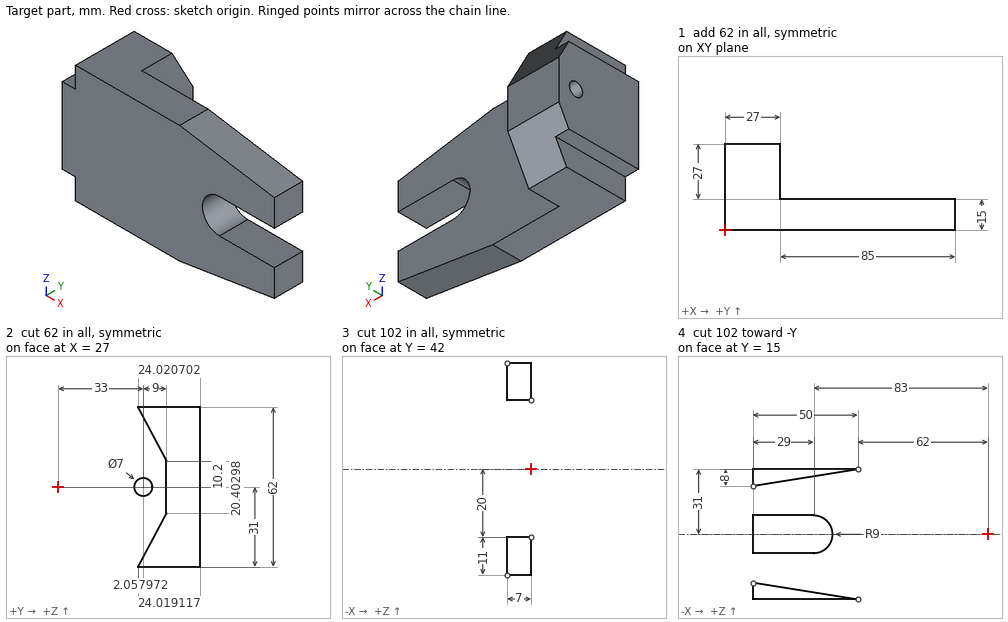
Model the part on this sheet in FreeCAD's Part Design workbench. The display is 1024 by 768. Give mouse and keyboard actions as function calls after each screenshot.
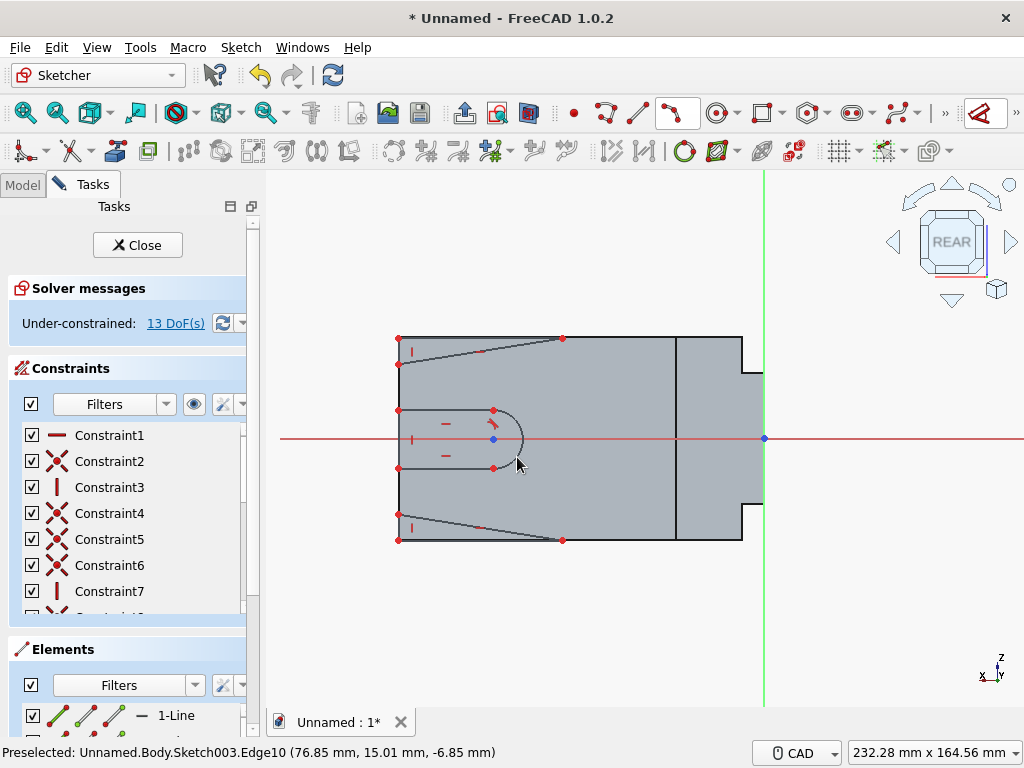
click(427, 469)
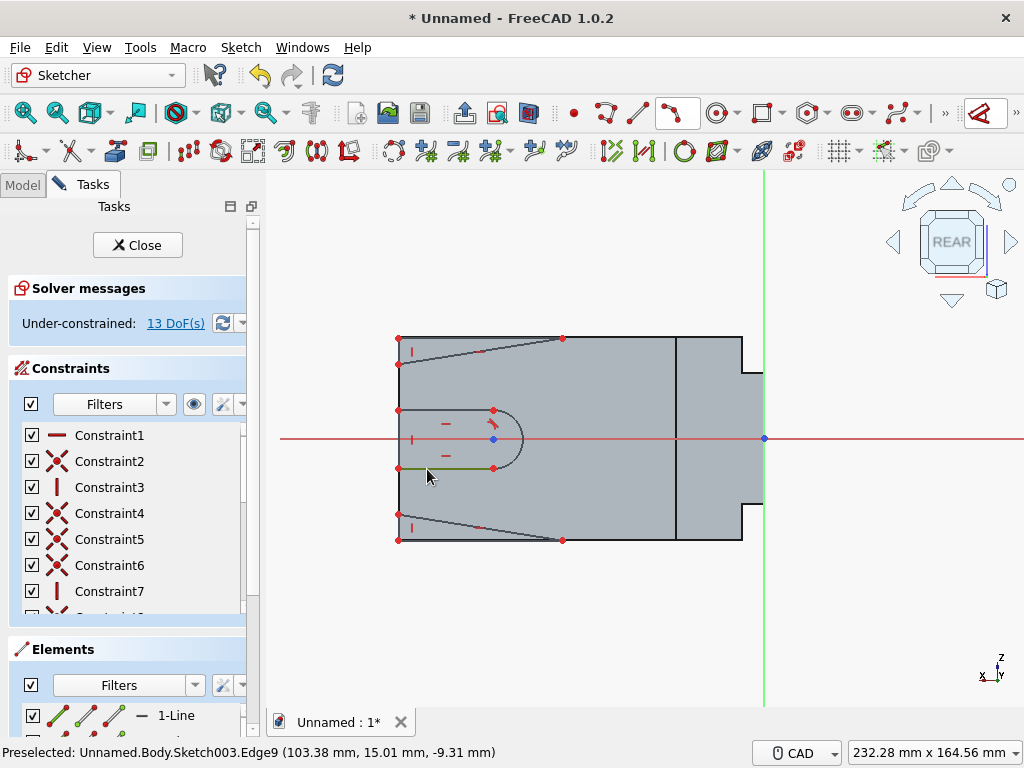
click(517, 457)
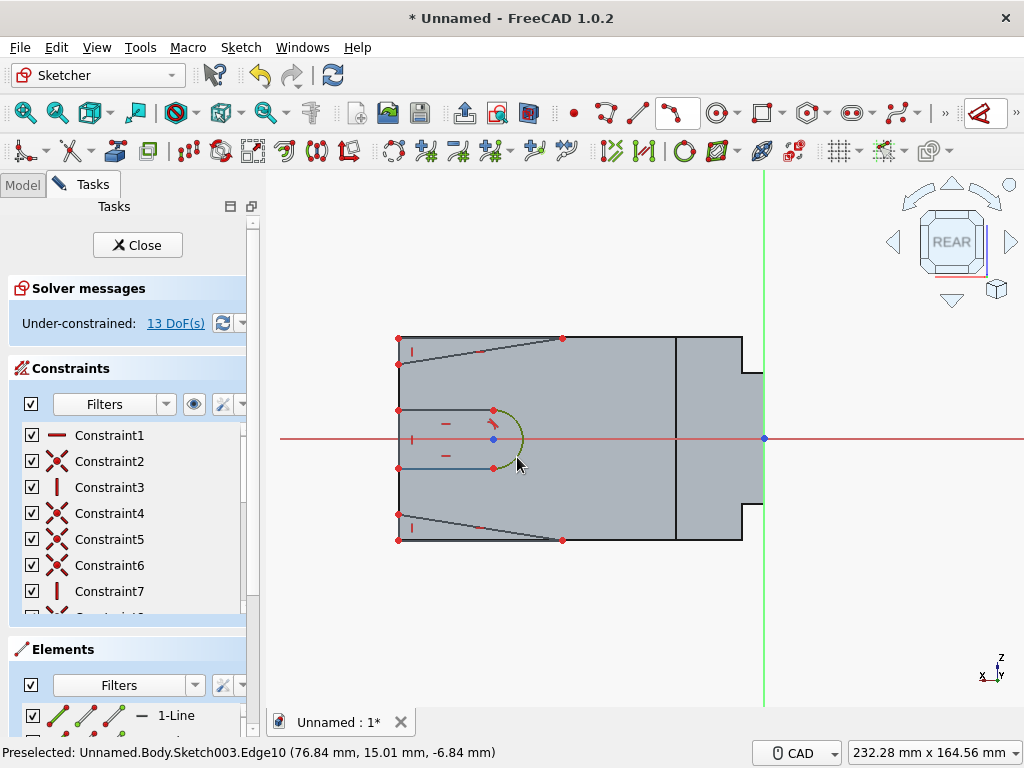
key(t)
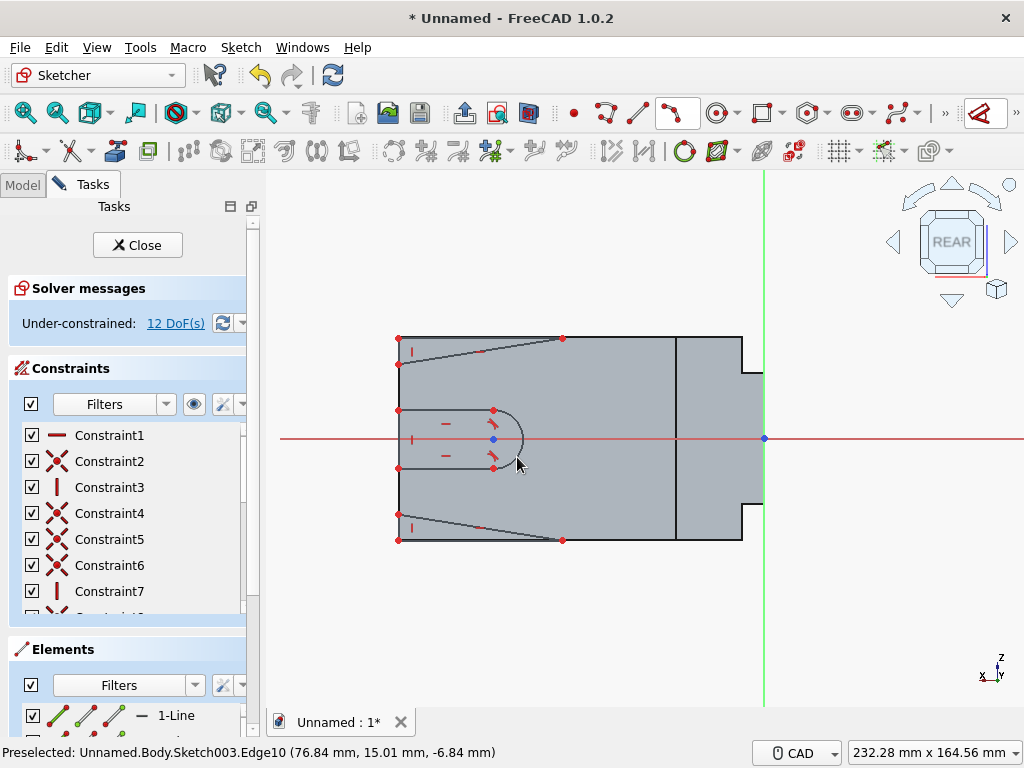
click(494, 439)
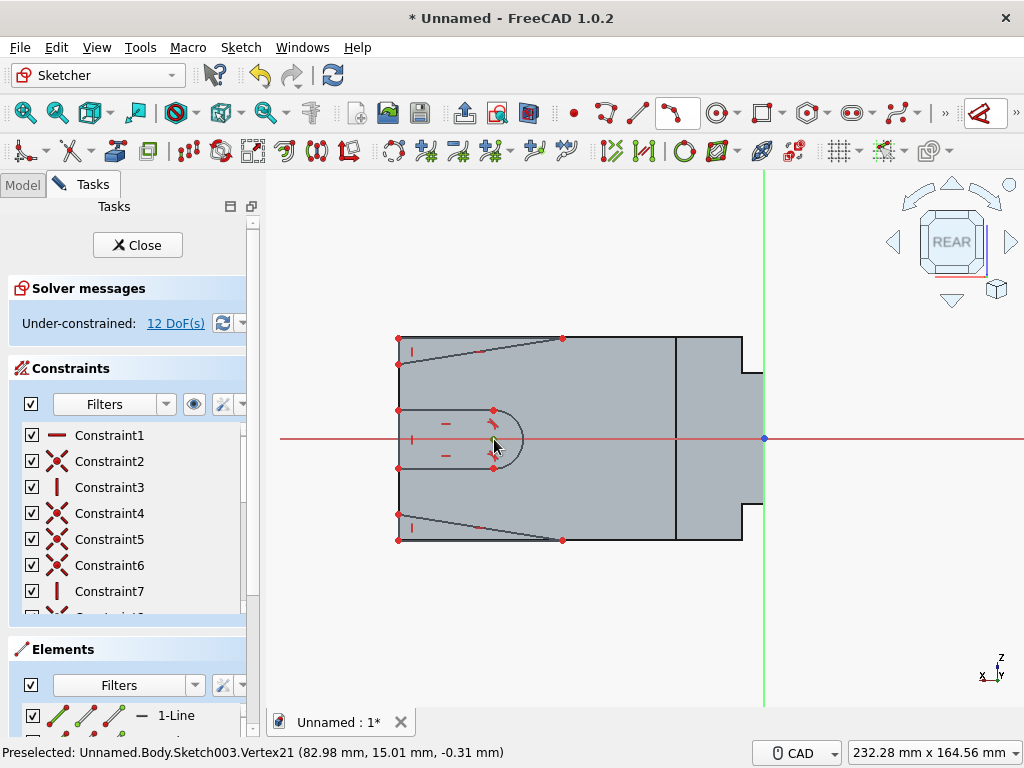
click(334, 439)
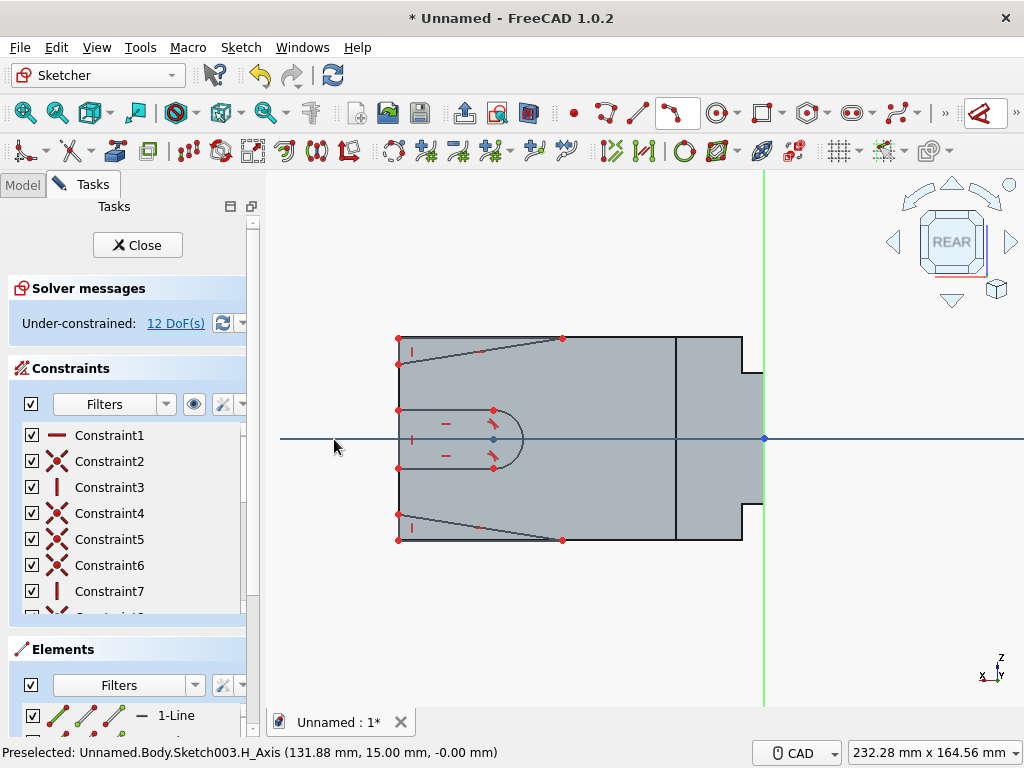
key(c)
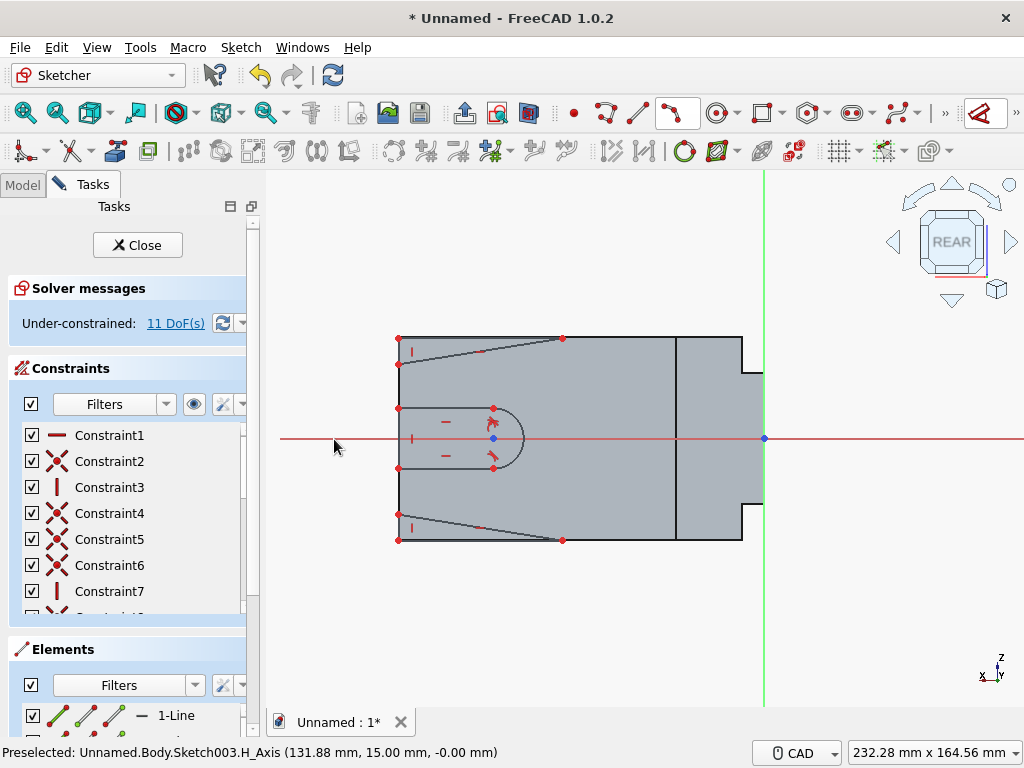
click(562, 338)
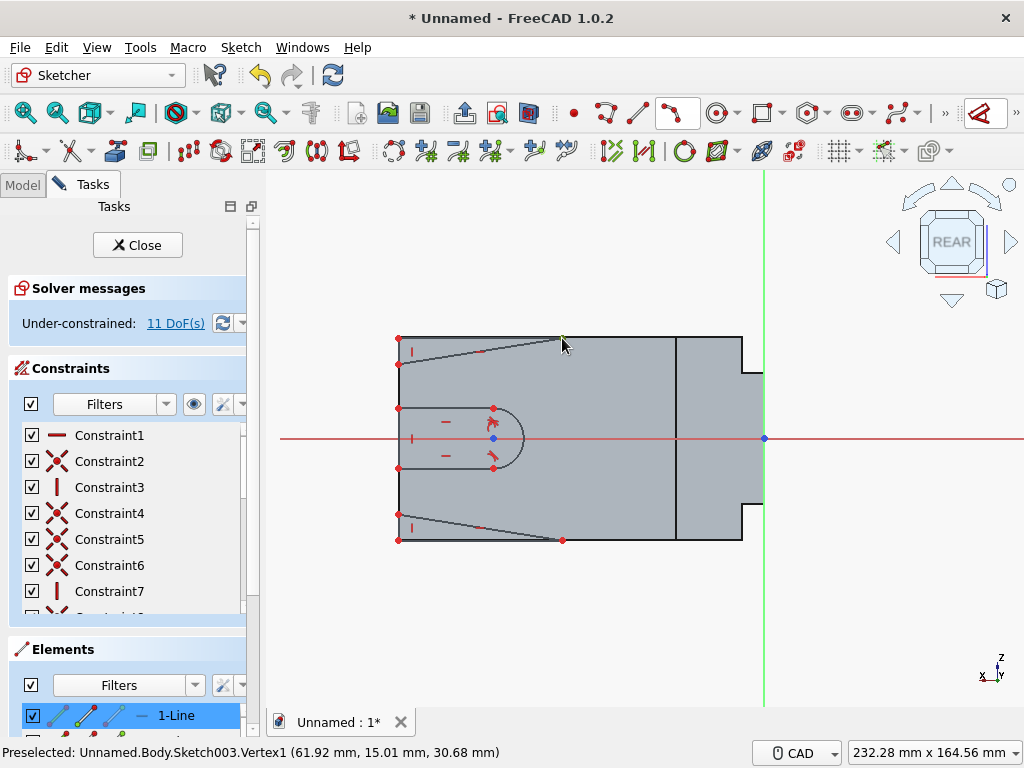
click(562, 541)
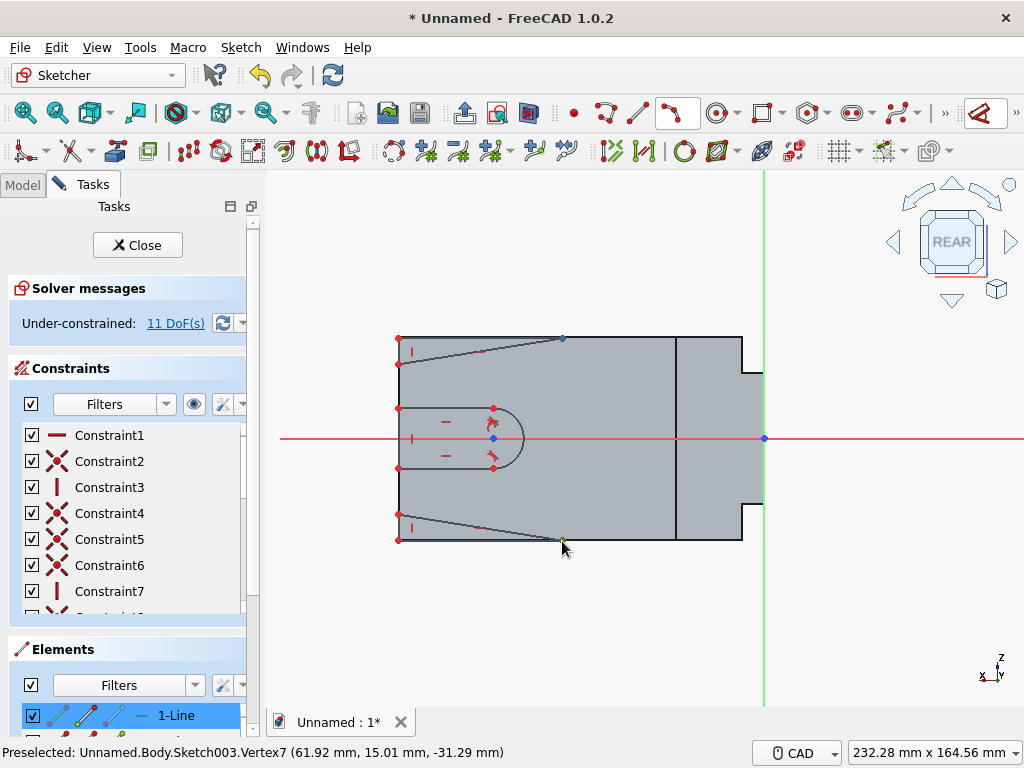
click(334, 439)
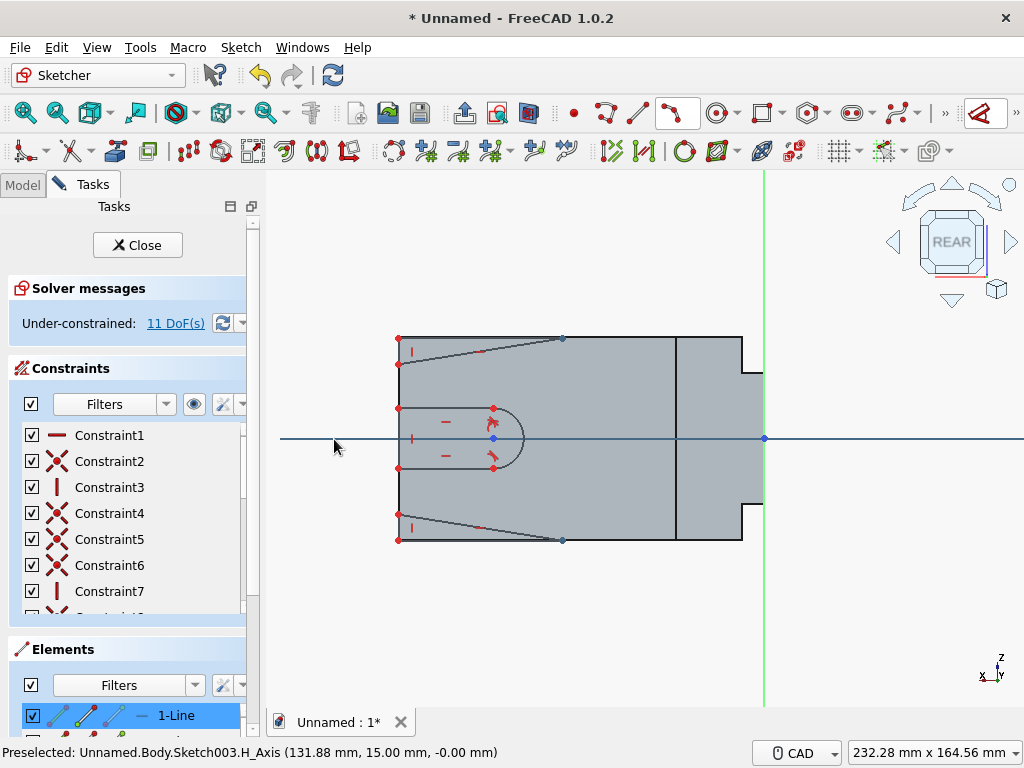
key(s)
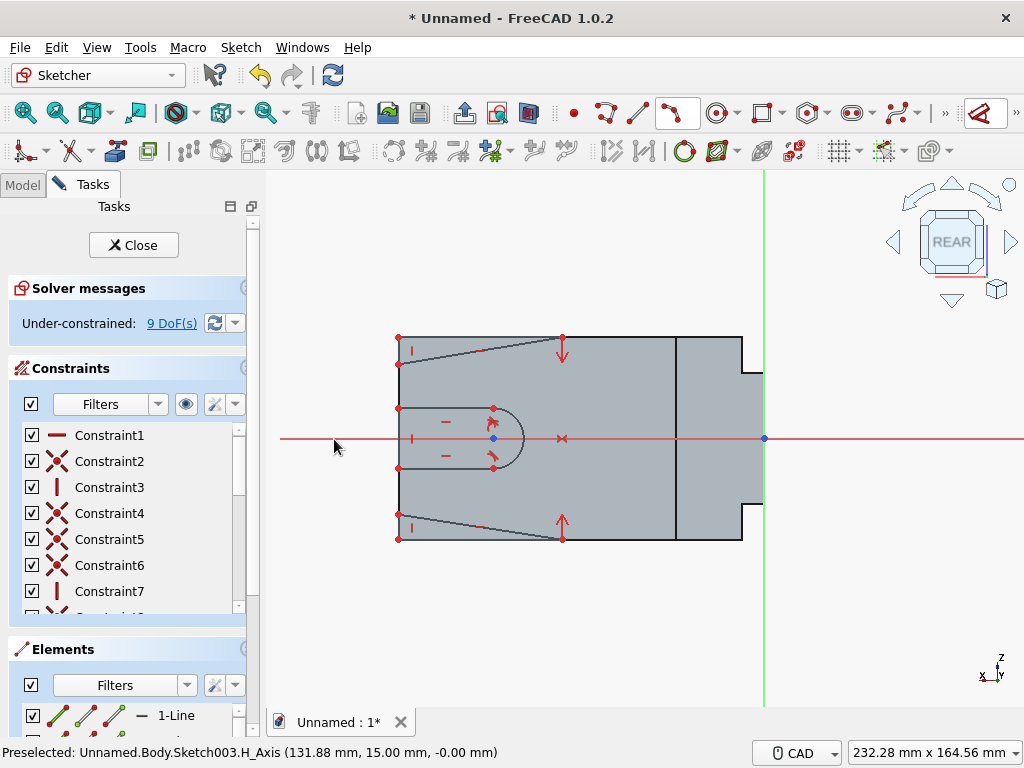
click(399, 364)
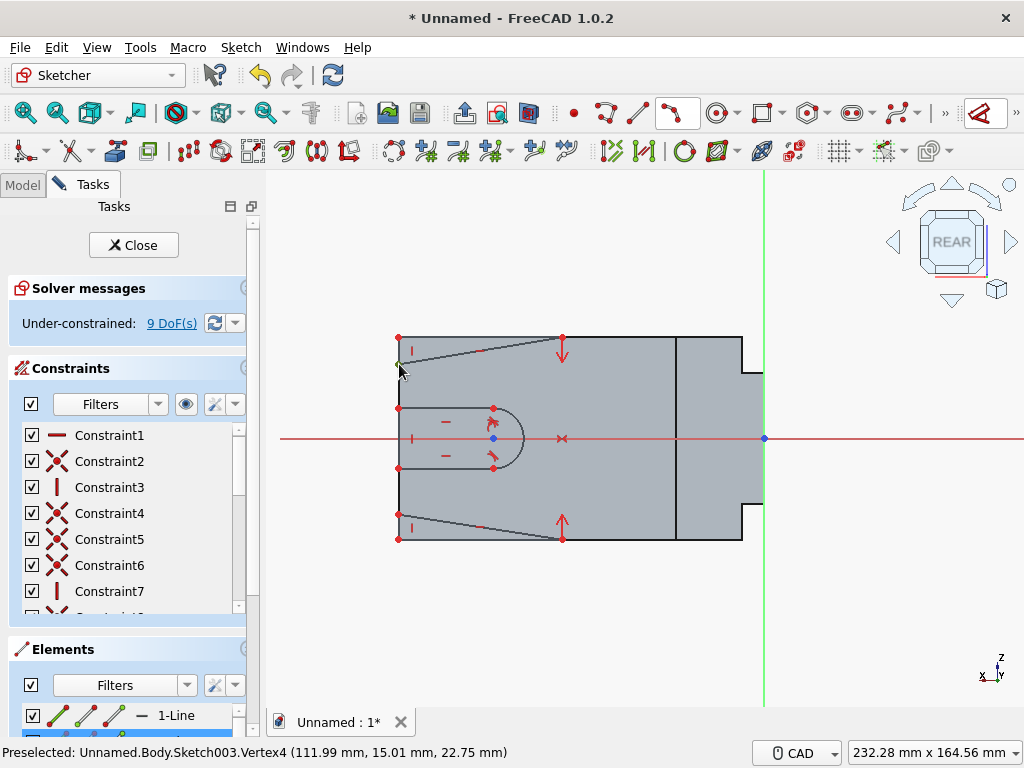
click(399, 515)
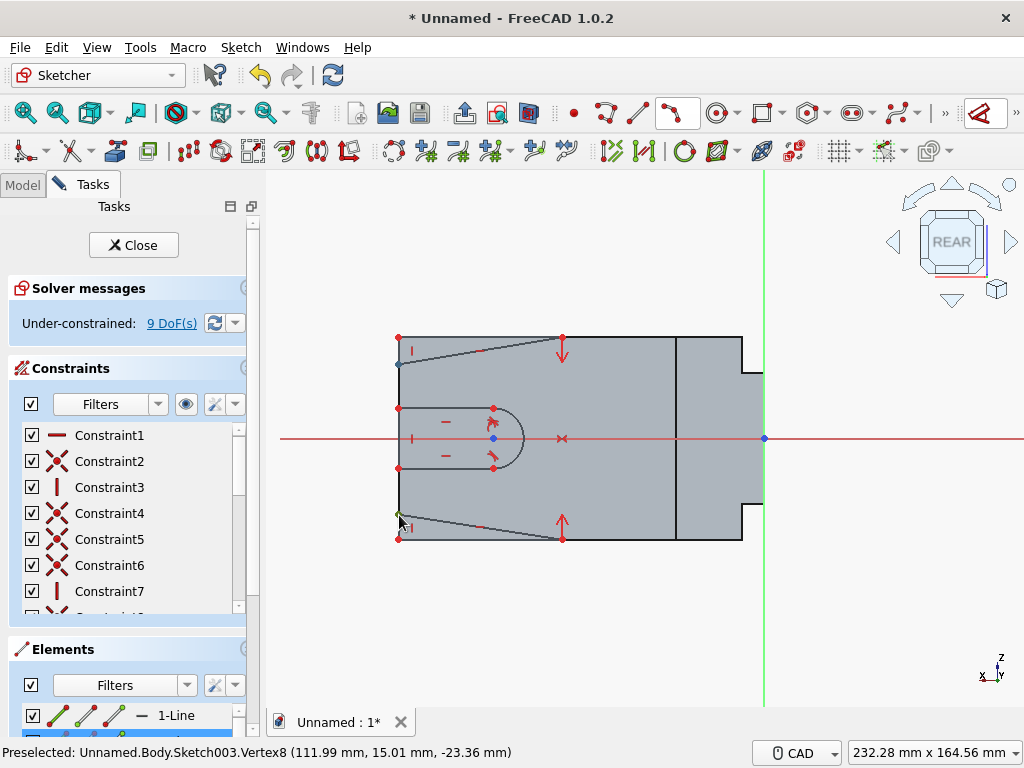
click(334, 439)